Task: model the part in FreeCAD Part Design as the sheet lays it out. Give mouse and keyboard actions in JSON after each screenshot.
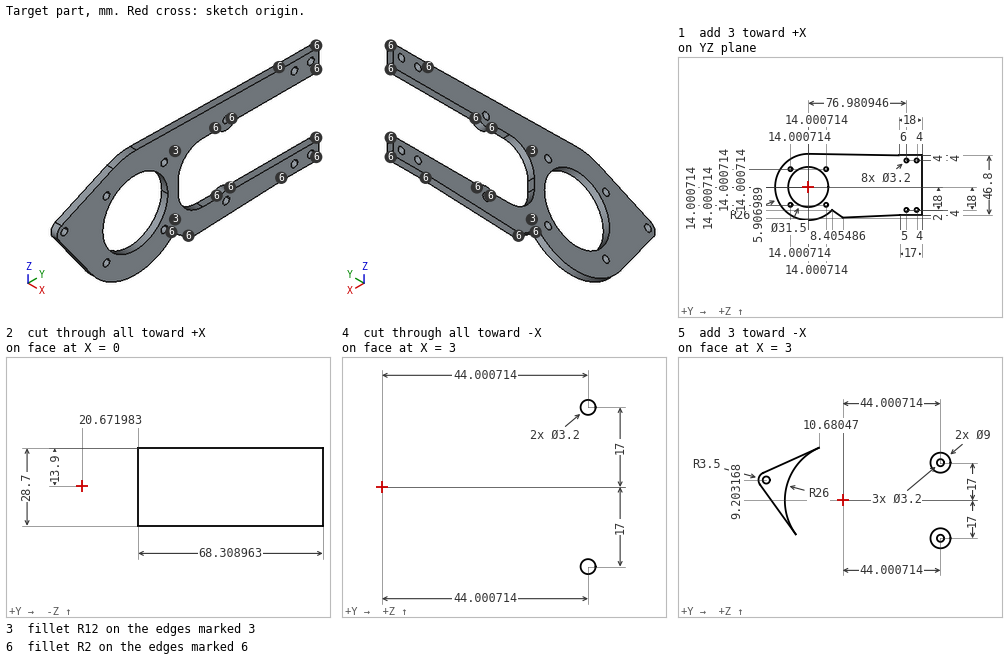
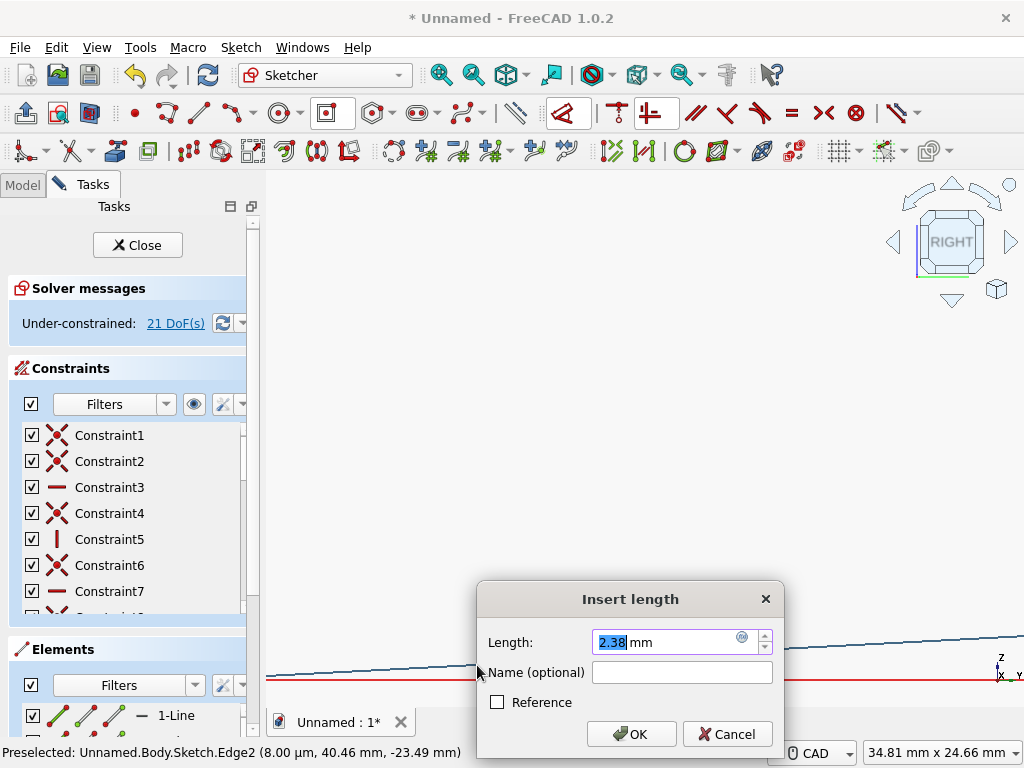
{"action": "type", "text": "2"}
{"action": "key", "text": "Return"}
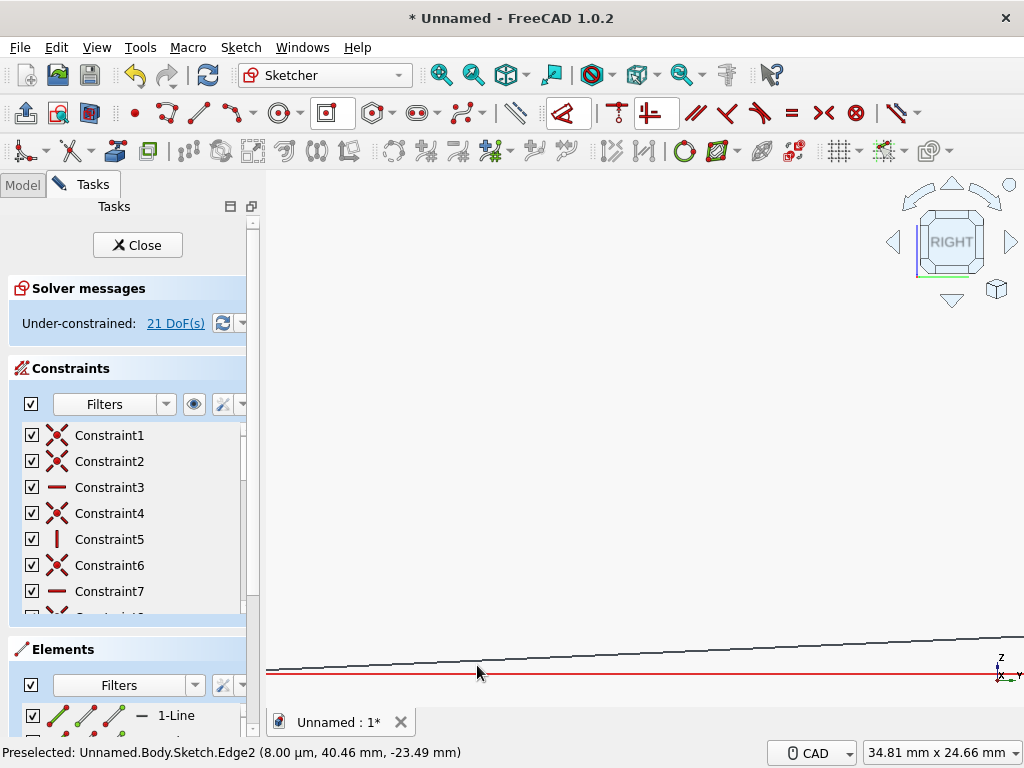
{"action": "scroll", "coordinate": [631, 499], "scroll_direction": "down", "scroll_amount": 9}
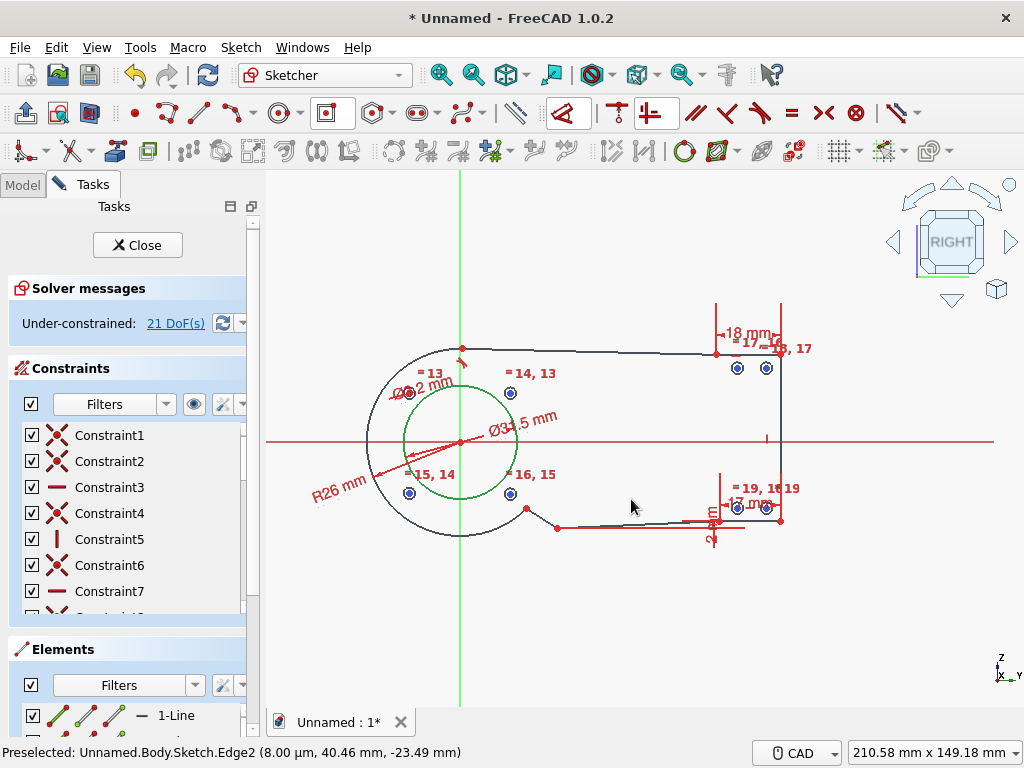
{"action": "left_click", "coordinate": [737, 508]}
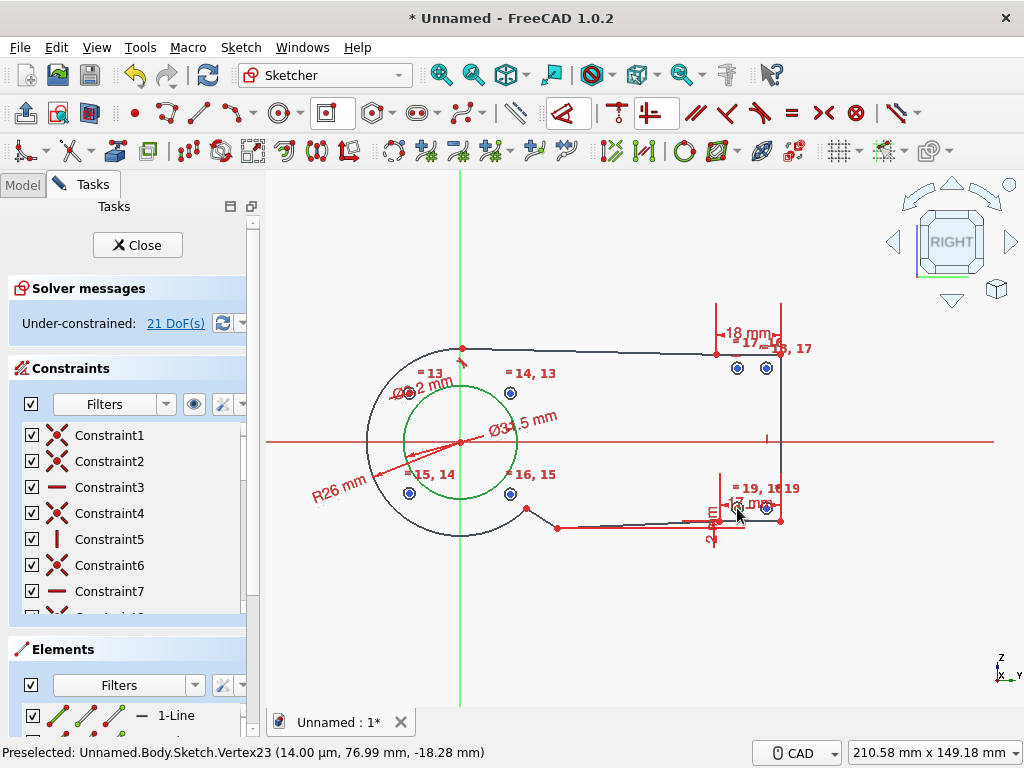
{"action": "key", "text": "i"}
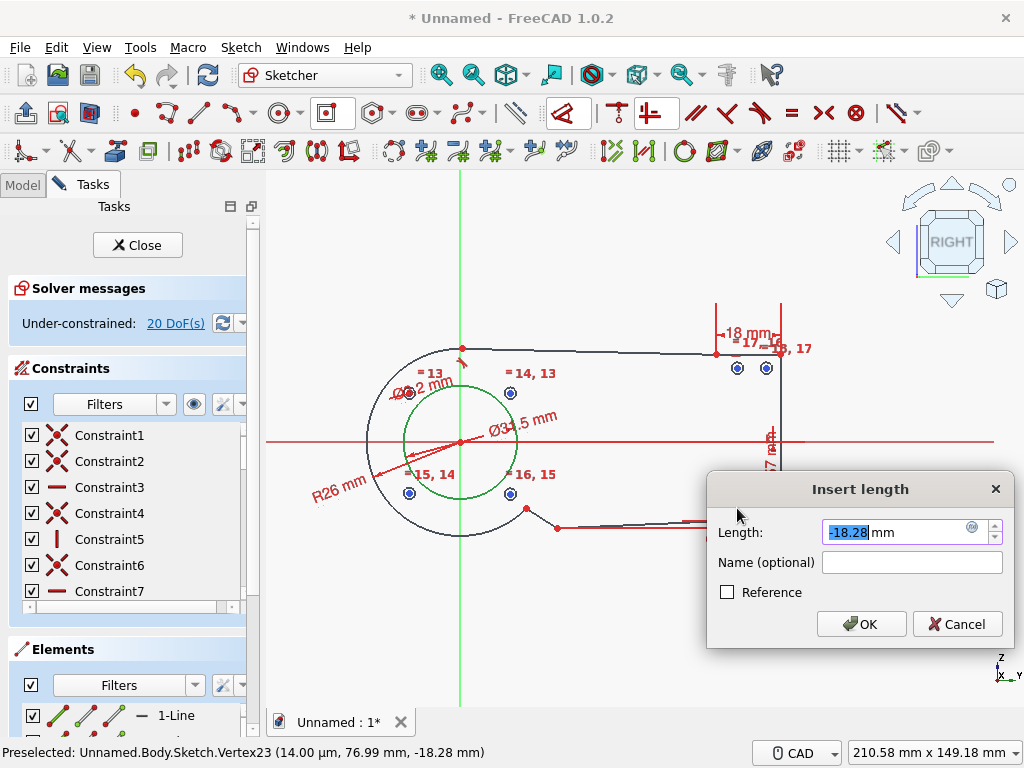
{"action": "type", "text": "-18"}
{"action": "key", "text": "Return"}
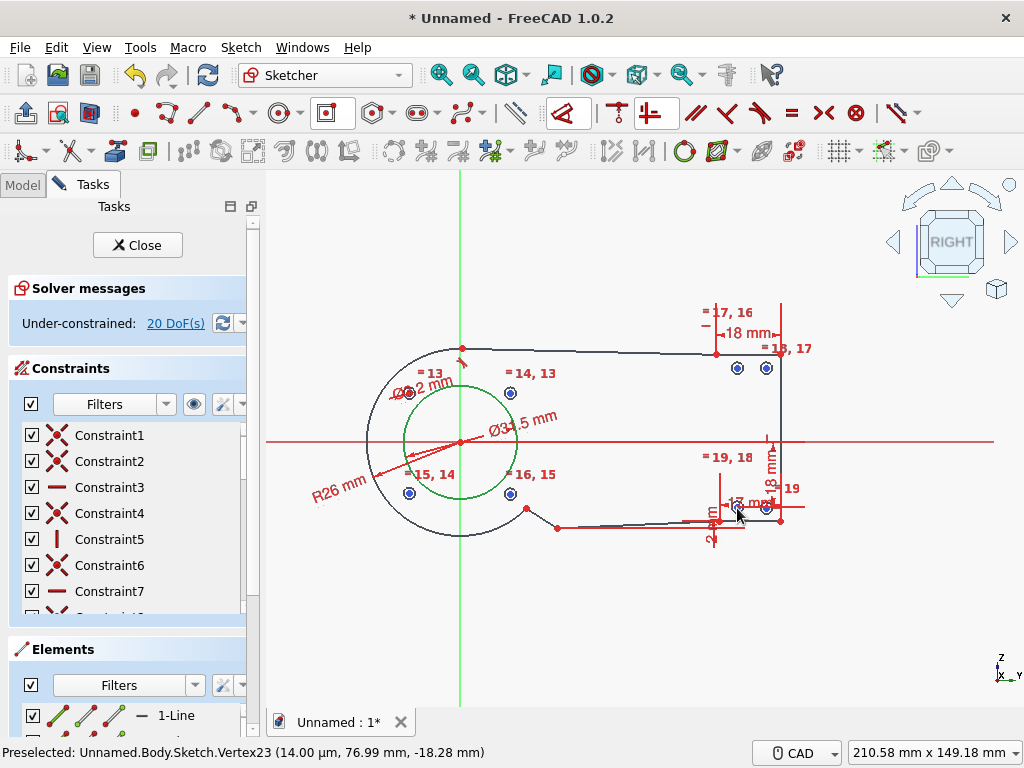
{"action": "left_click", "coordinate": [766, 508]}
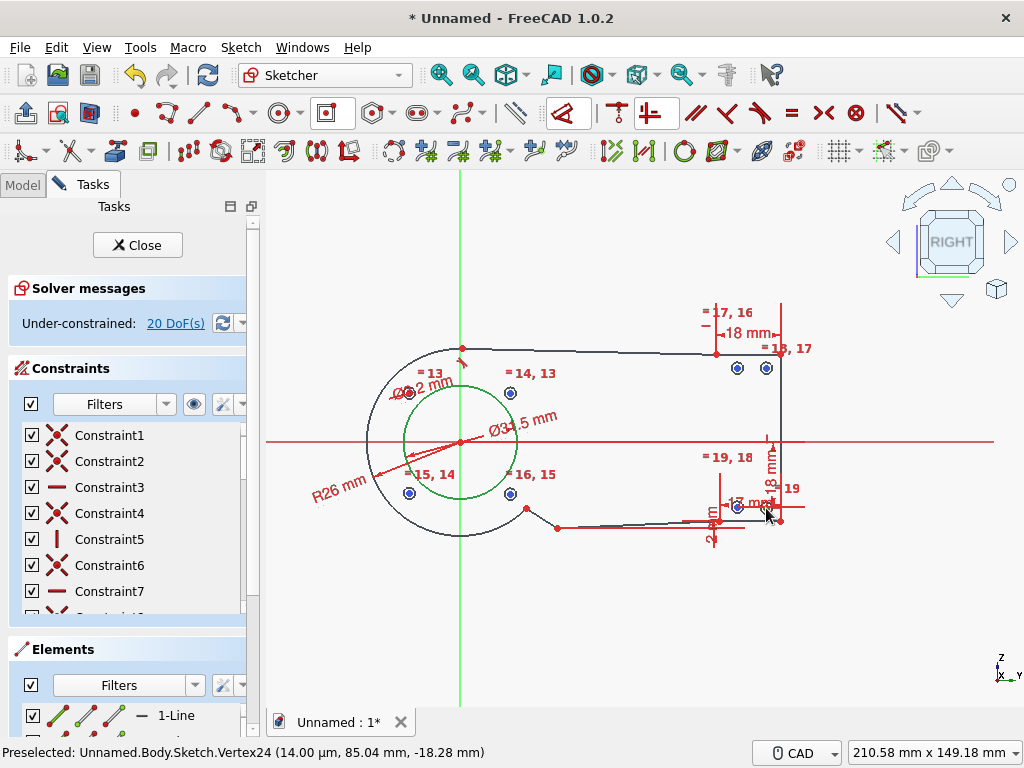
{"action": "key", "text": "i"}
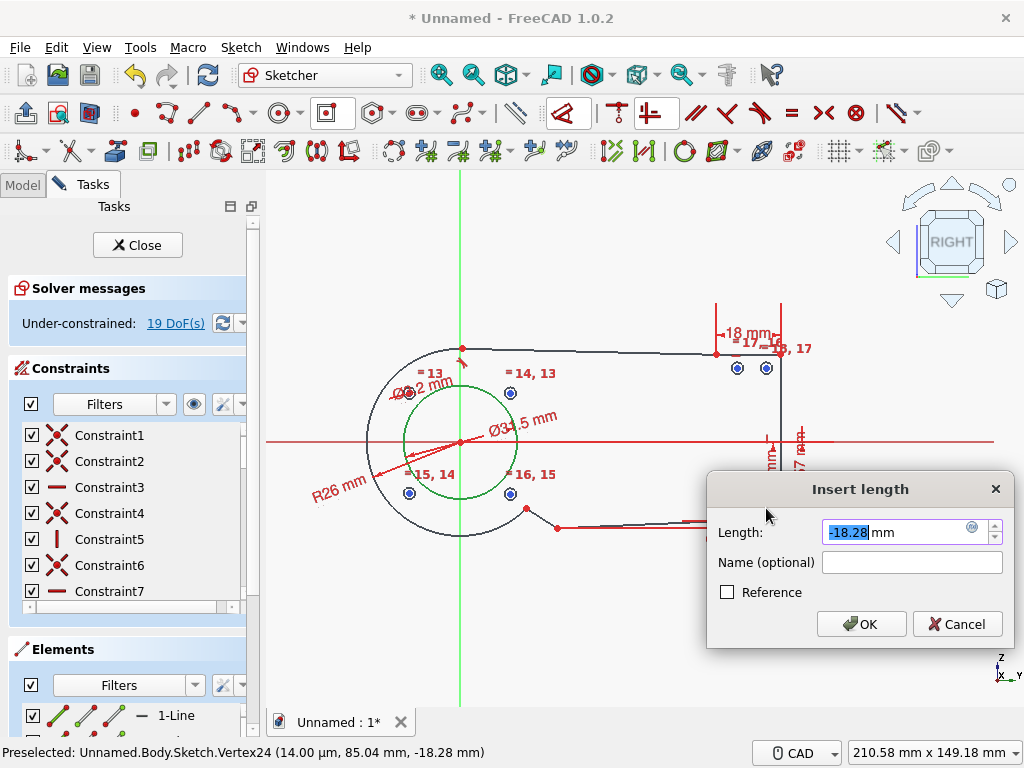
{"action": "type", "text": "-18"}
{"action": "key", "text": "Return"}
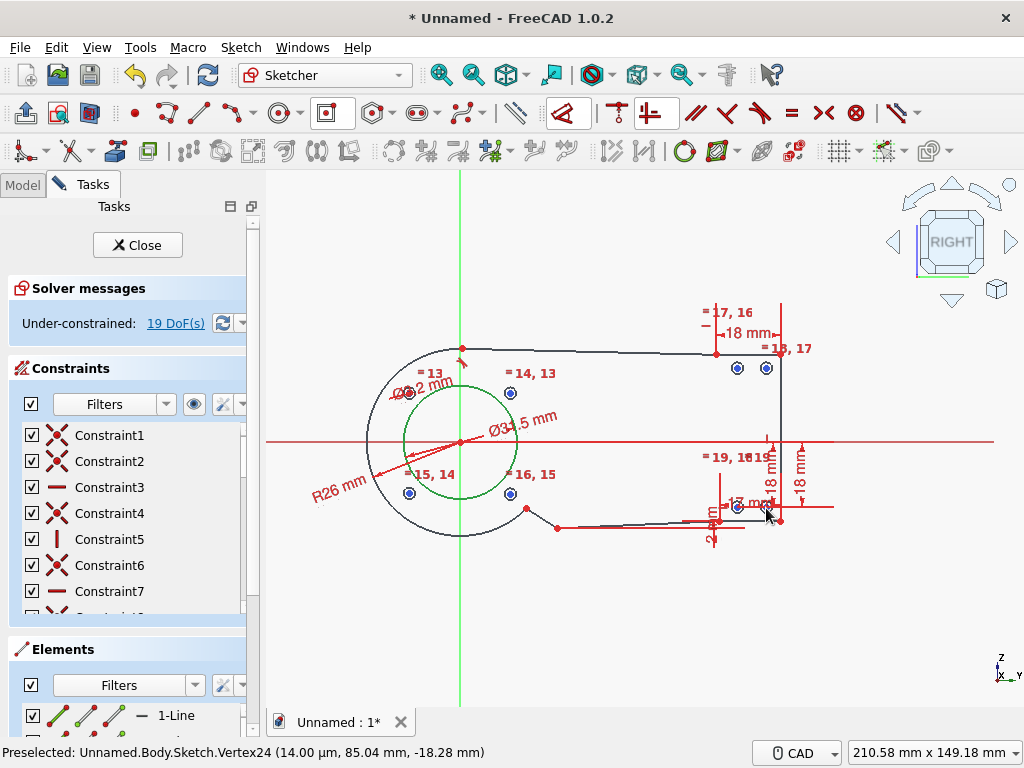
{"action": "scroll", "coordinate": [716, 355], "scroll_direction": "up", "scroll_amount": 4}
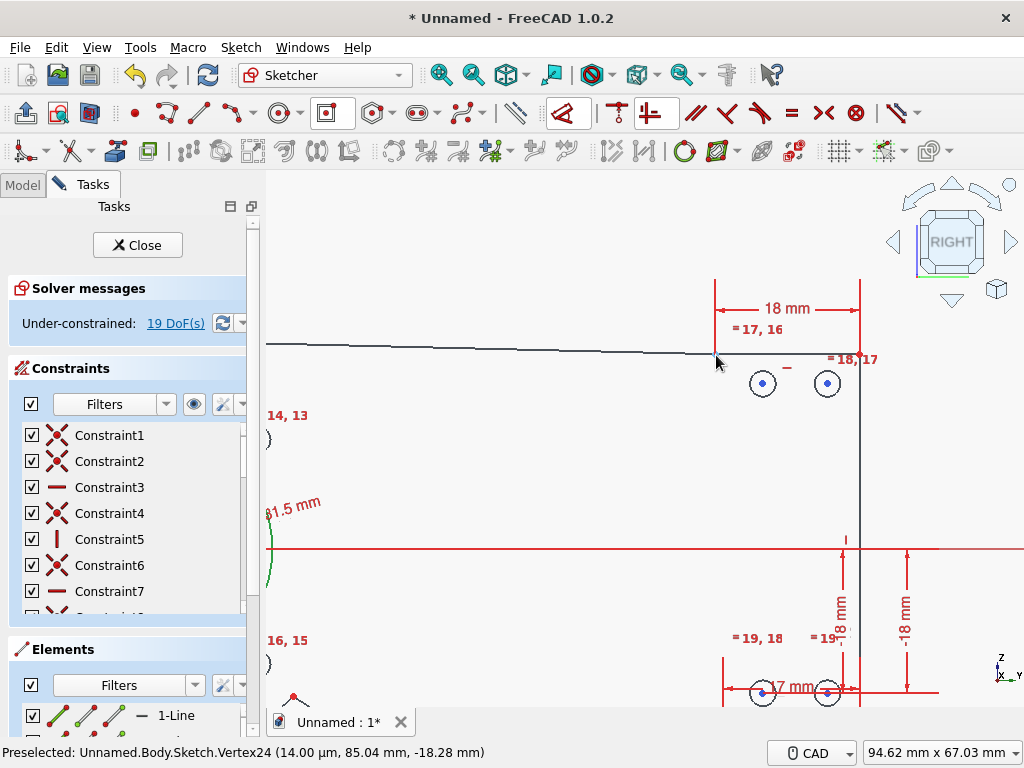
{"action": "left_click", "coordinate": [715, 354]}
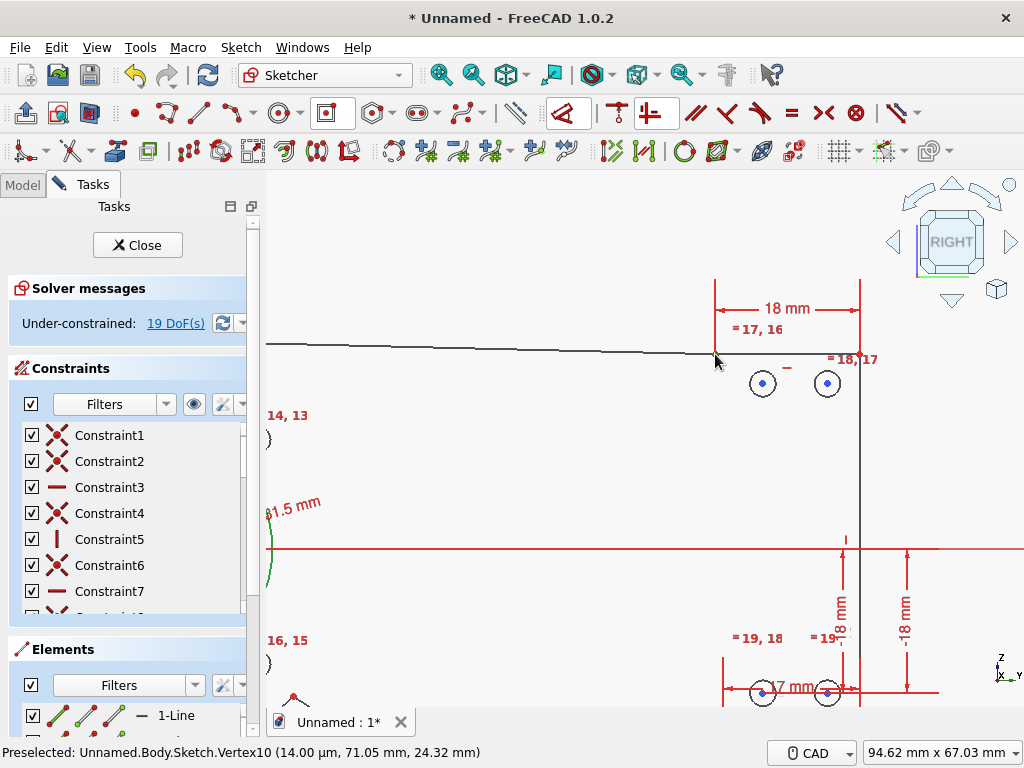
{"action": "left_click", "coordinate": [763, 384]}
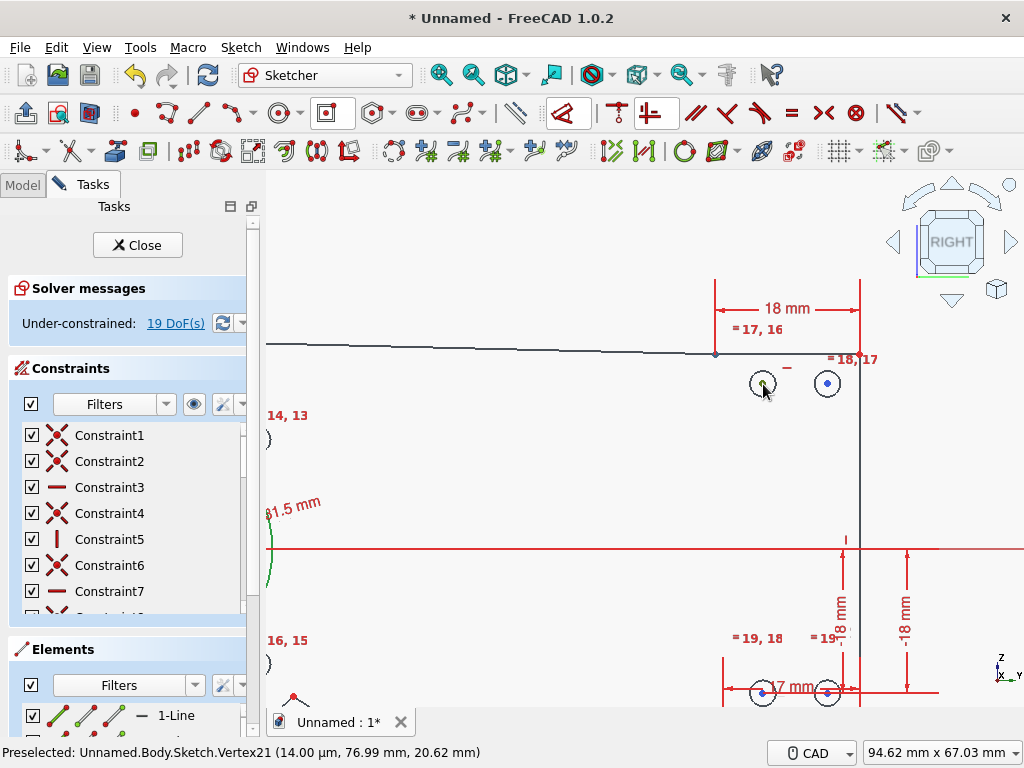
{"action": "left_click", "coordinate": [586, 114]}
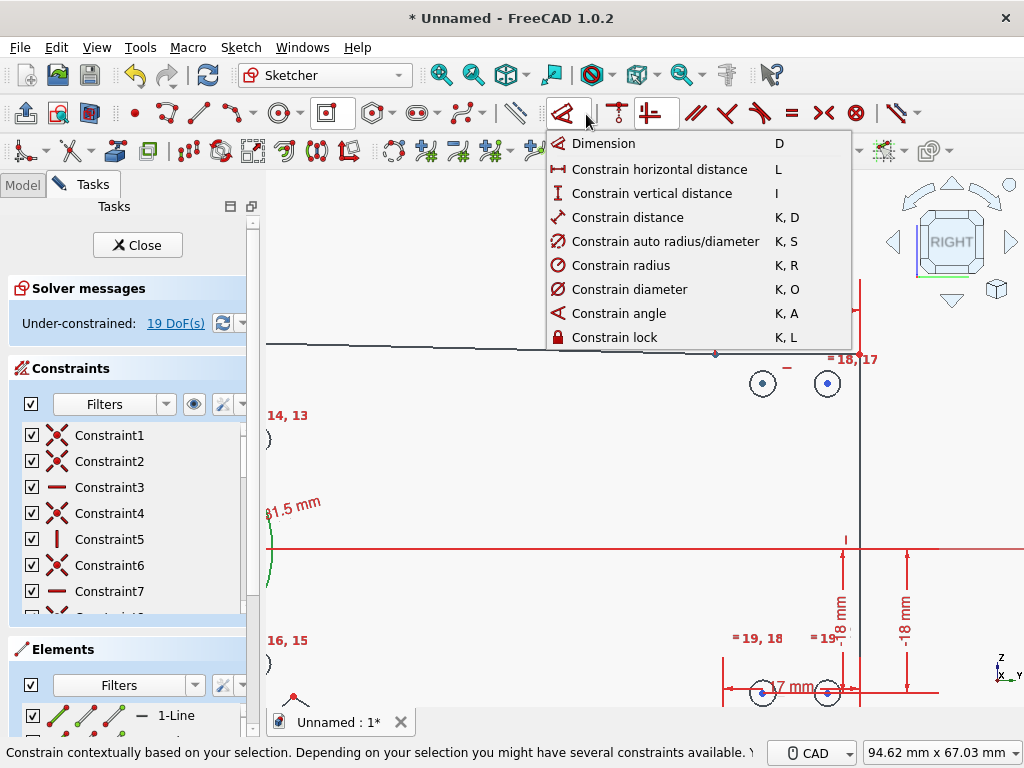
{"action": "left_click", "coordinate": [699, 169]}